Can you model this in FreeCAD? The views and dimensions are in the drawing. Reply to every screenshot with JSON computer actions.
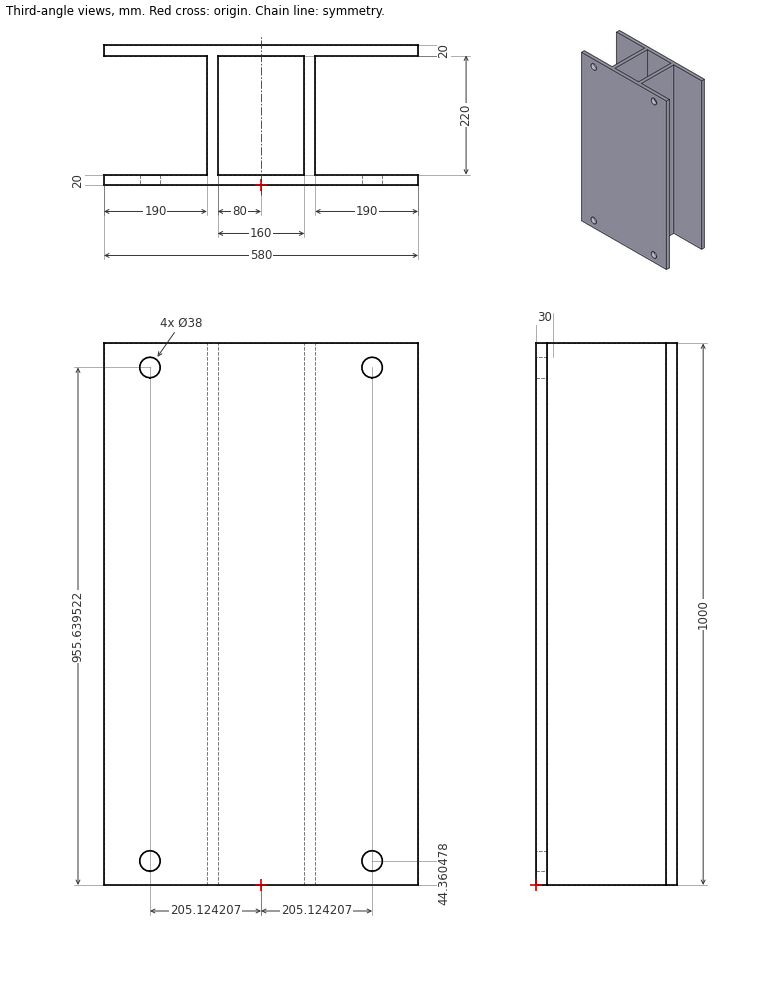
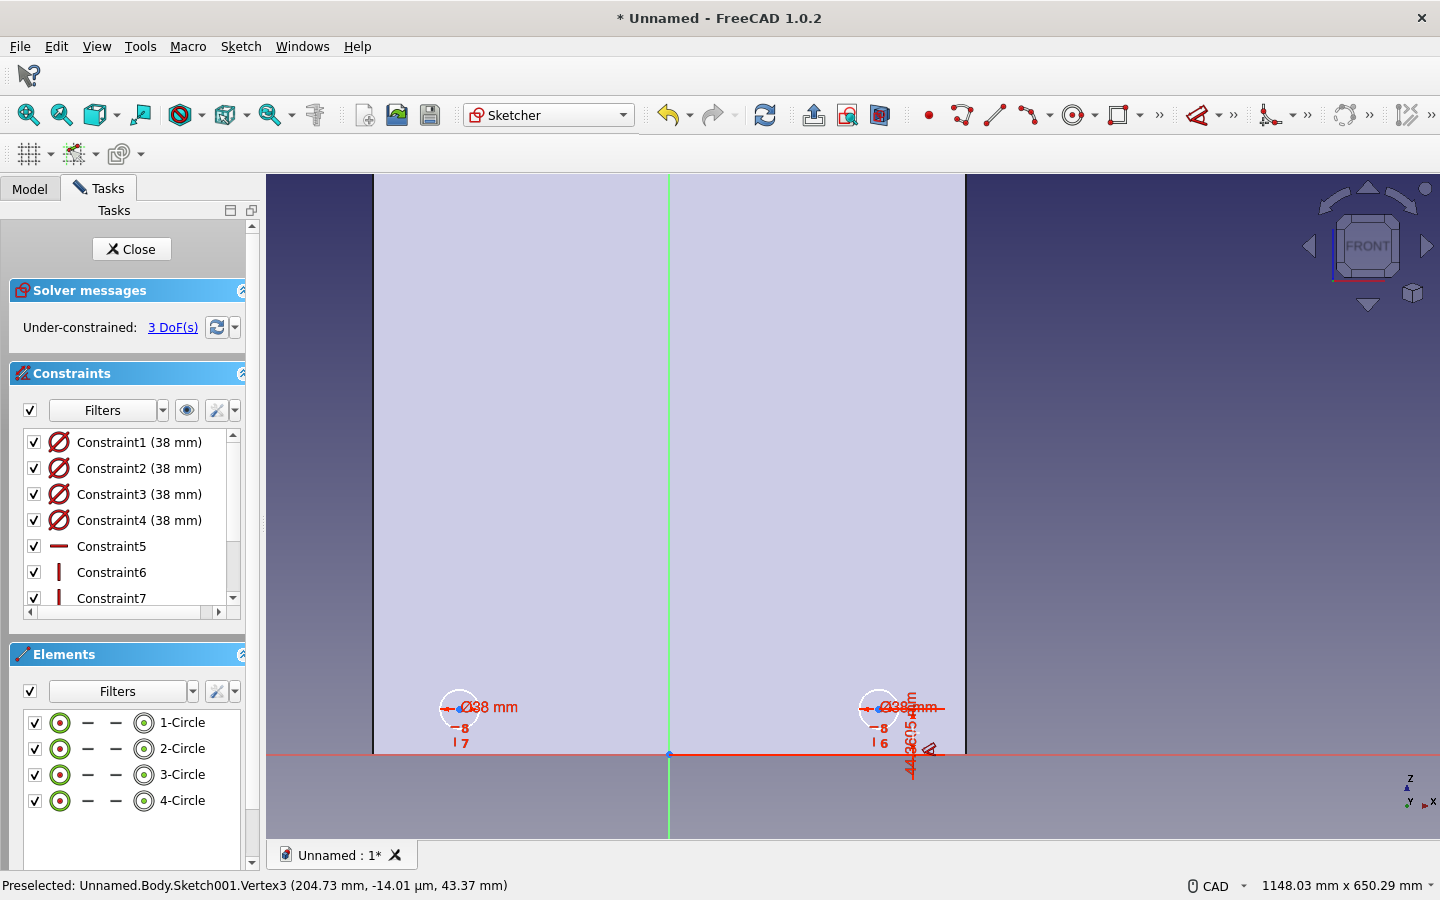
{"action": "scroll", "coordinate": [878, 711], "scroll_direction": "down", "scroll_amount": 4}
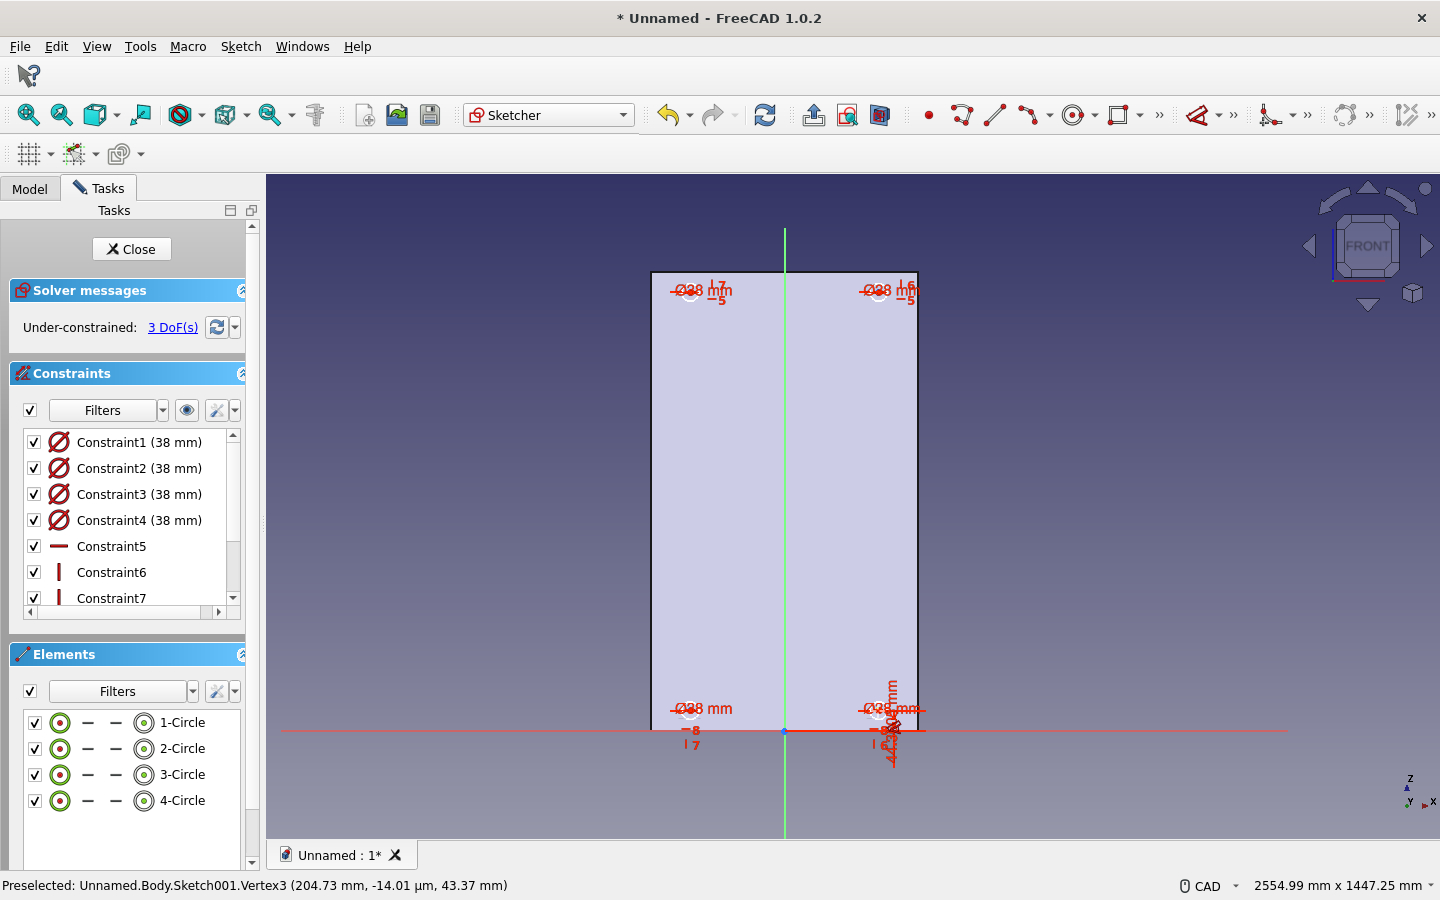
{"action": "left_click", "coordinate": [690, 292]}
{"action": "left_click", "coordinate": [737, 765]}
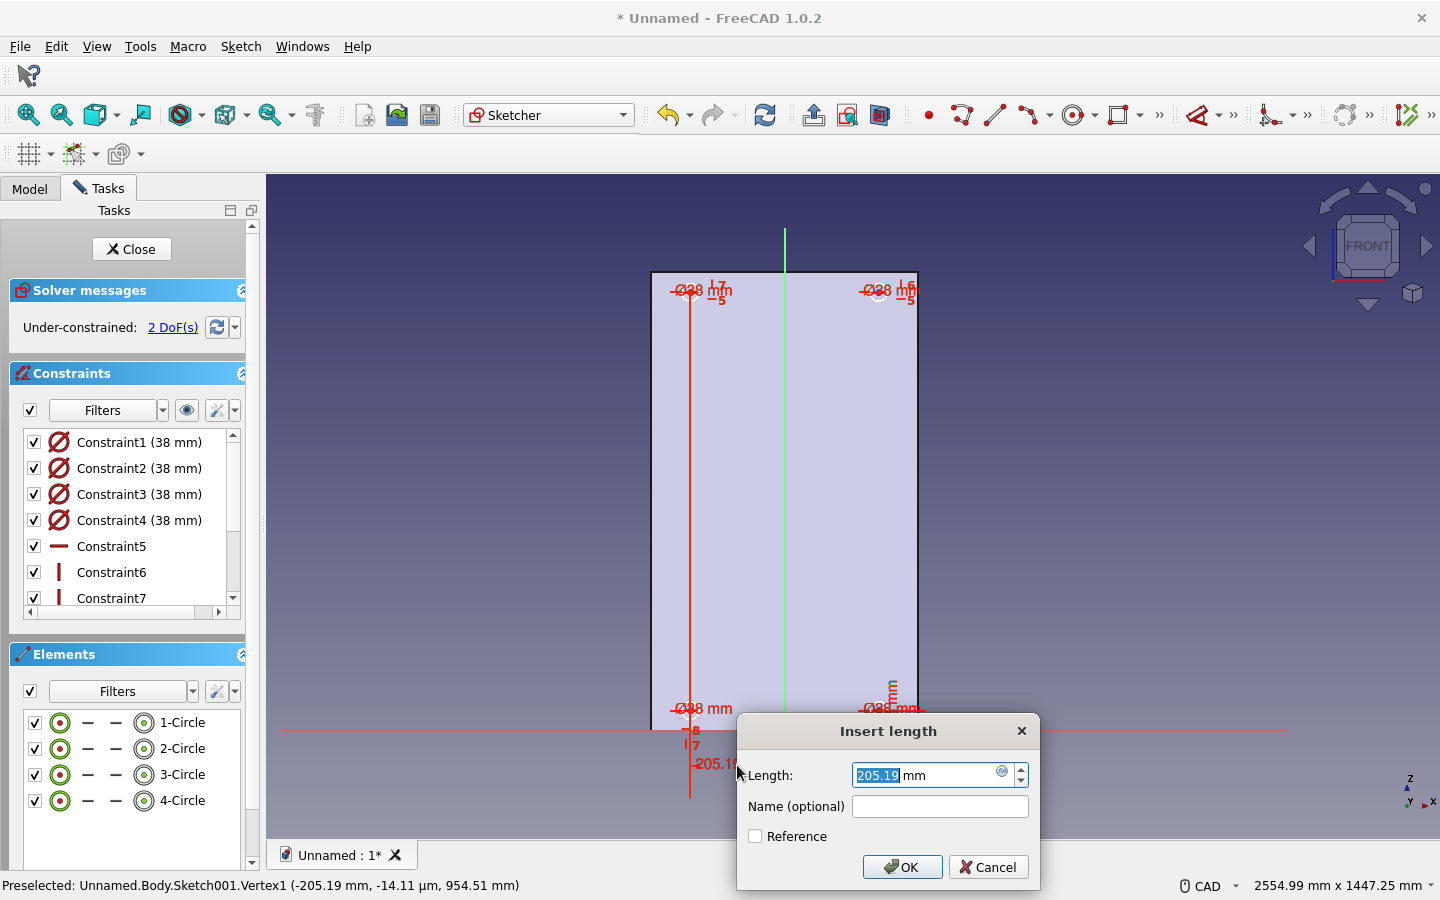
{"action": "type", "text": "205.124207"}
{"action": "key", "text": "Return"}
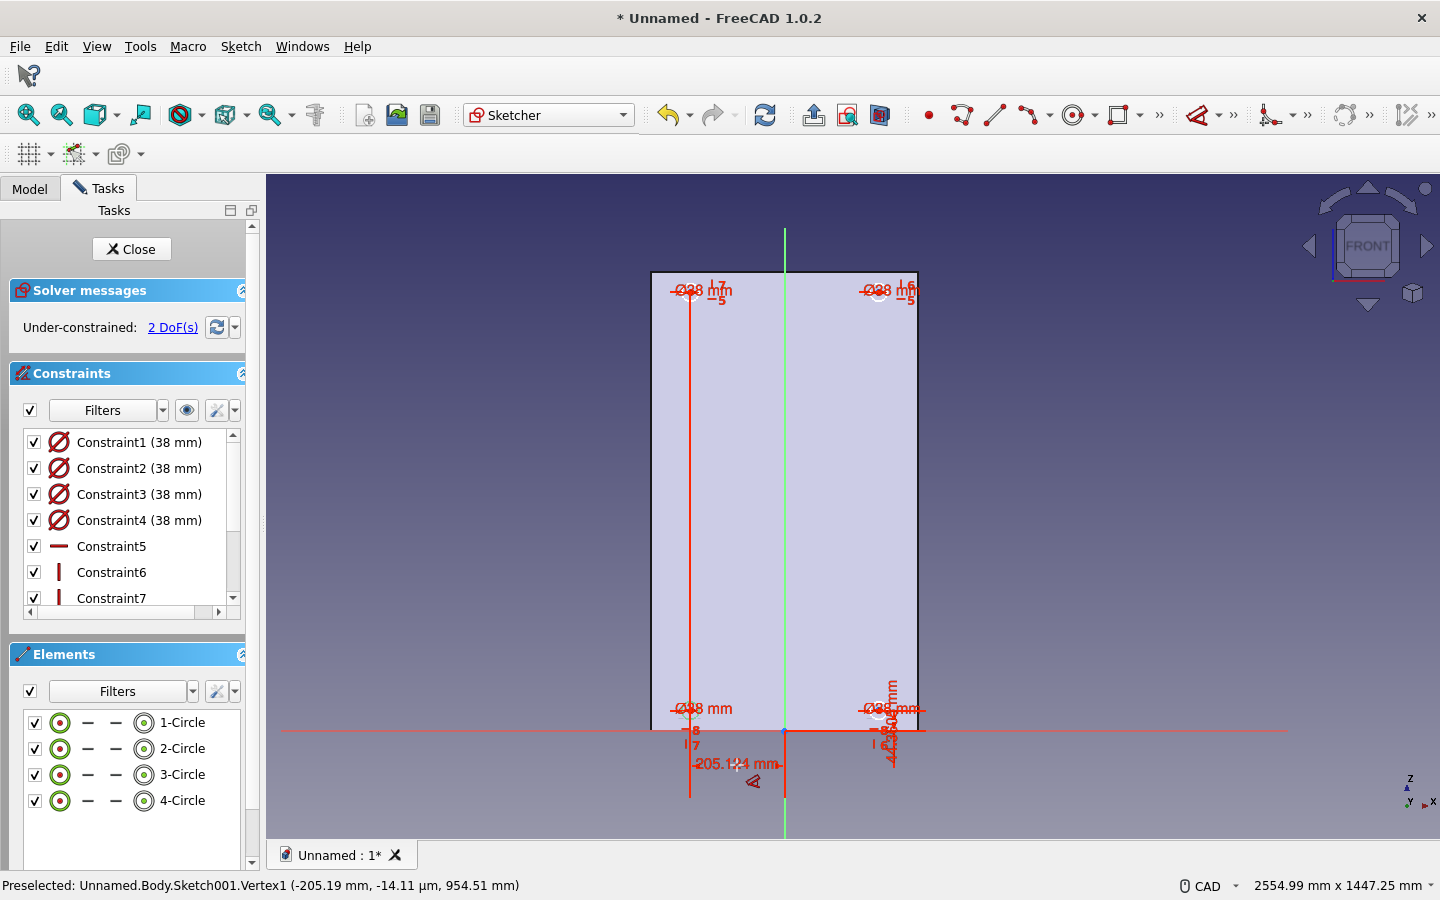
{"action": "left_click", "coordinate": [690, 292]}
{"action": "left_click", "coordinate": [656, 512]}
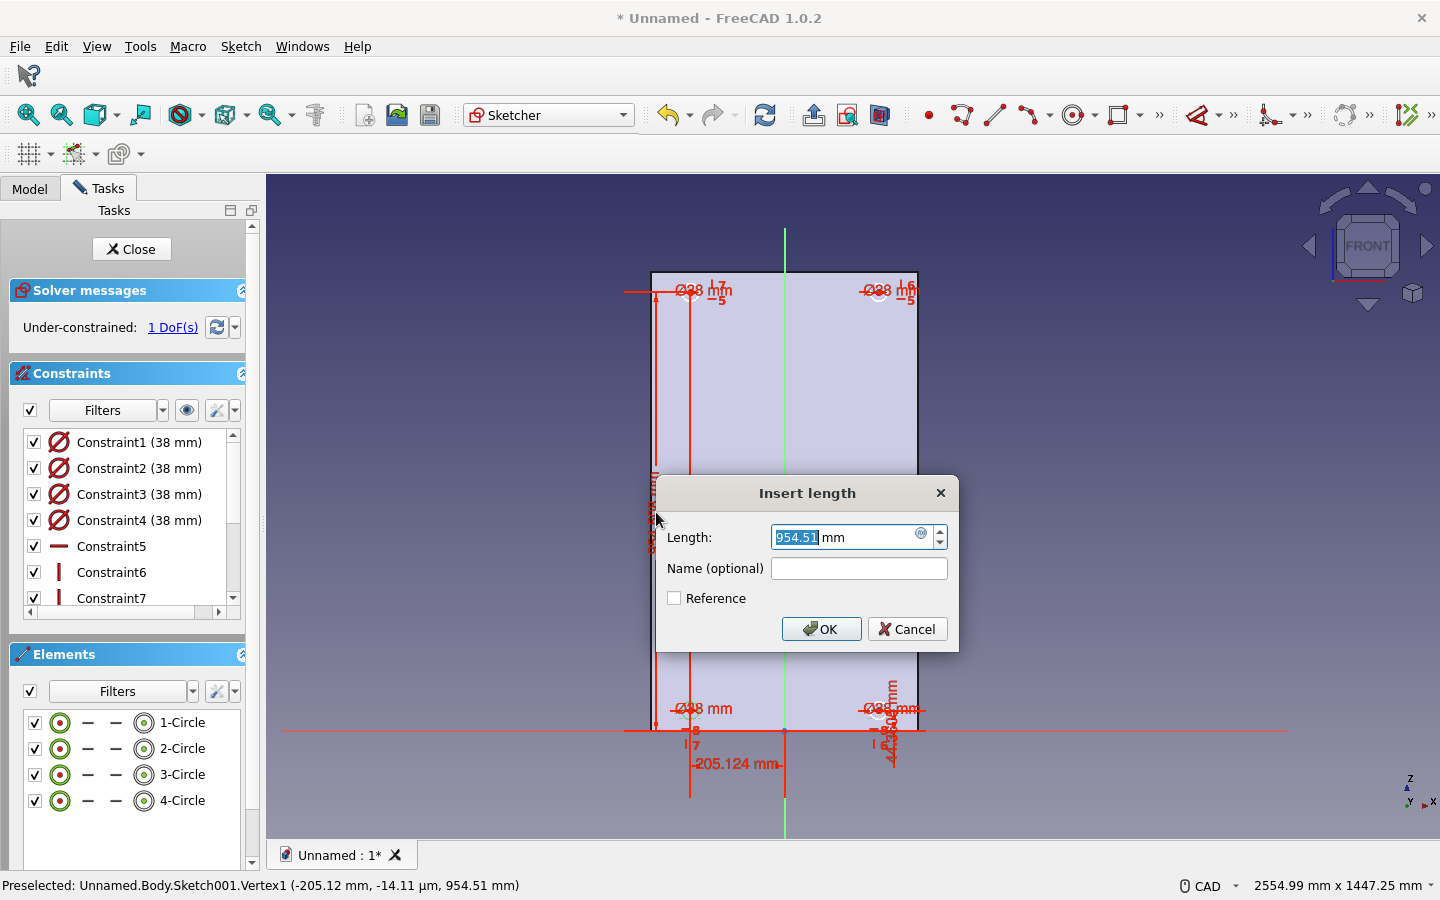
{"action": "type", "text": "955.639522"}
{"action": "key", "text": "Return"}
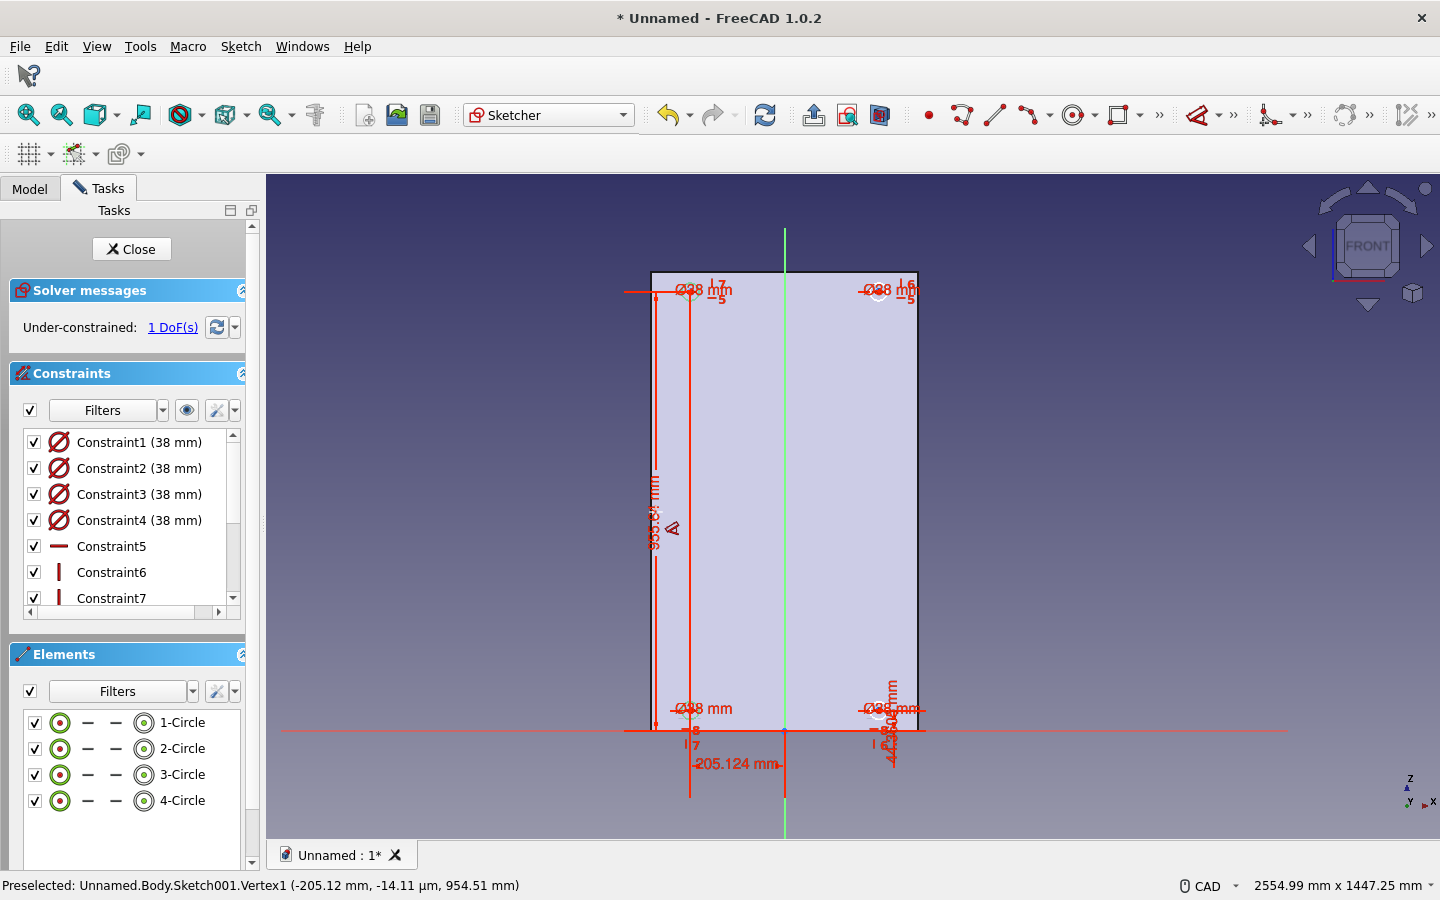
{"action": "left_click", "coordinate": [879, 292]}
{"action": "left_click", "coordinate": [832, 765]}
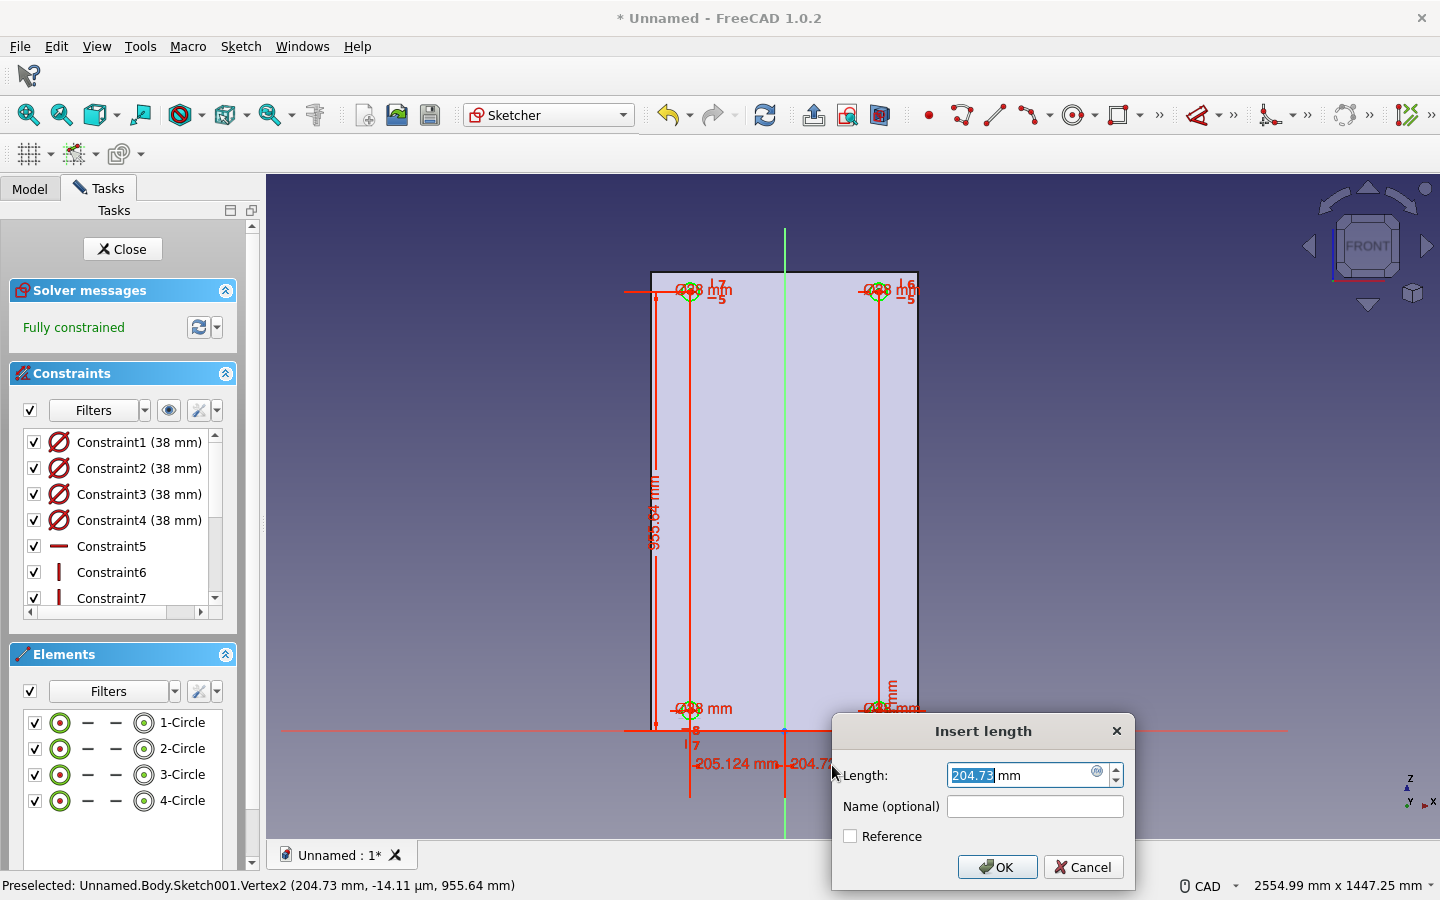
{"action": "type", "text": "205.124207"}
{"action": "key", "text": "Return"}
{"action": "key", "text": "Escape"}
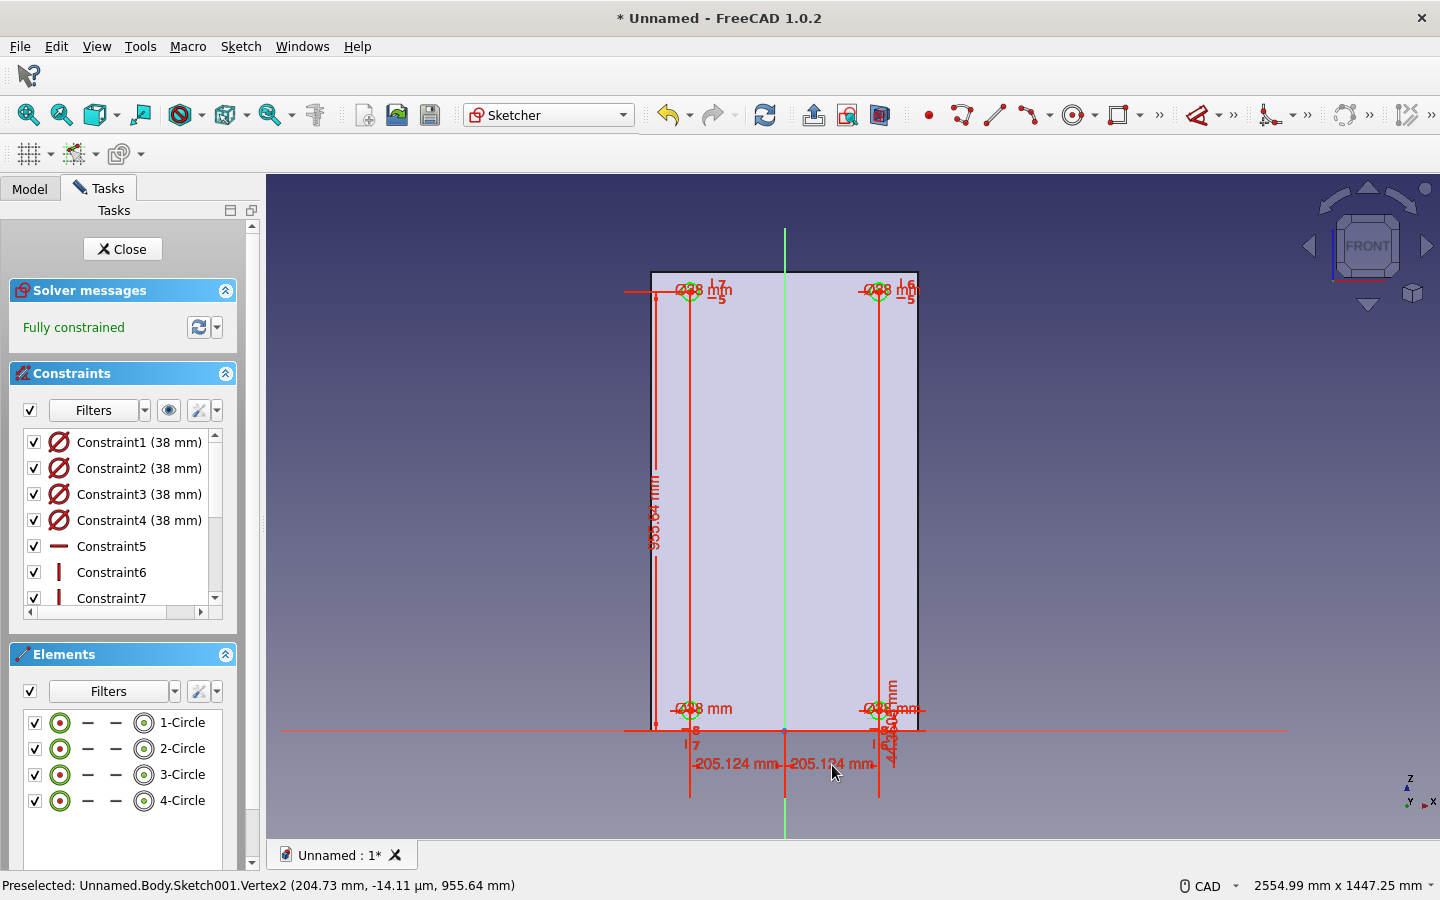
{"action": "left_click", "coordinate": [123, 249]}